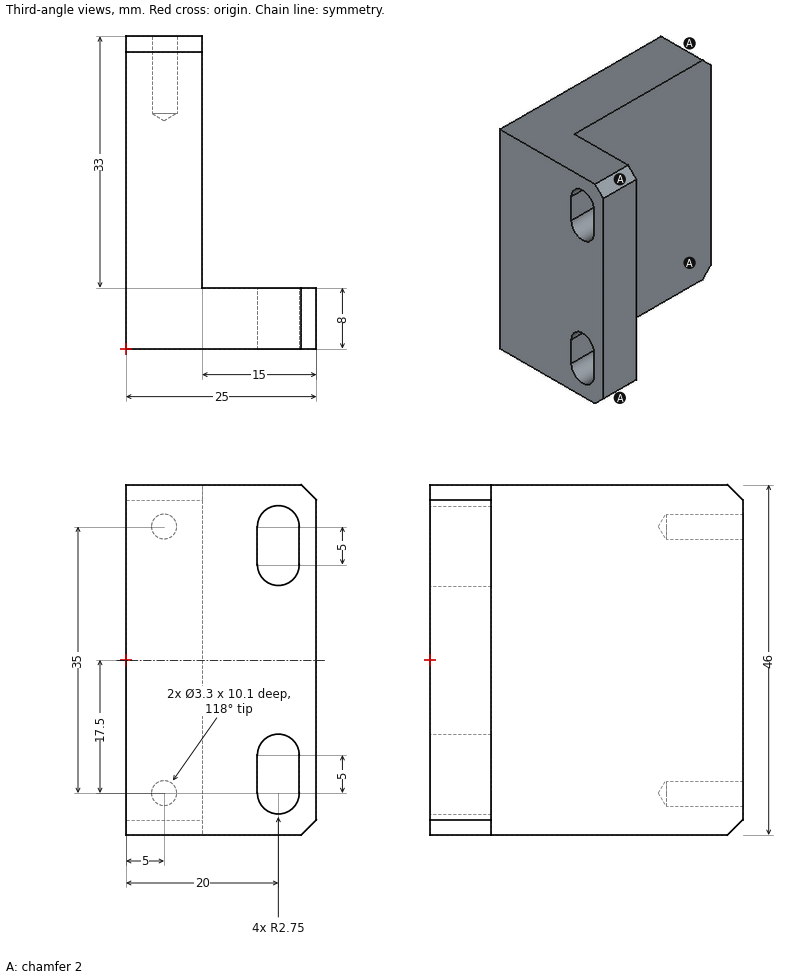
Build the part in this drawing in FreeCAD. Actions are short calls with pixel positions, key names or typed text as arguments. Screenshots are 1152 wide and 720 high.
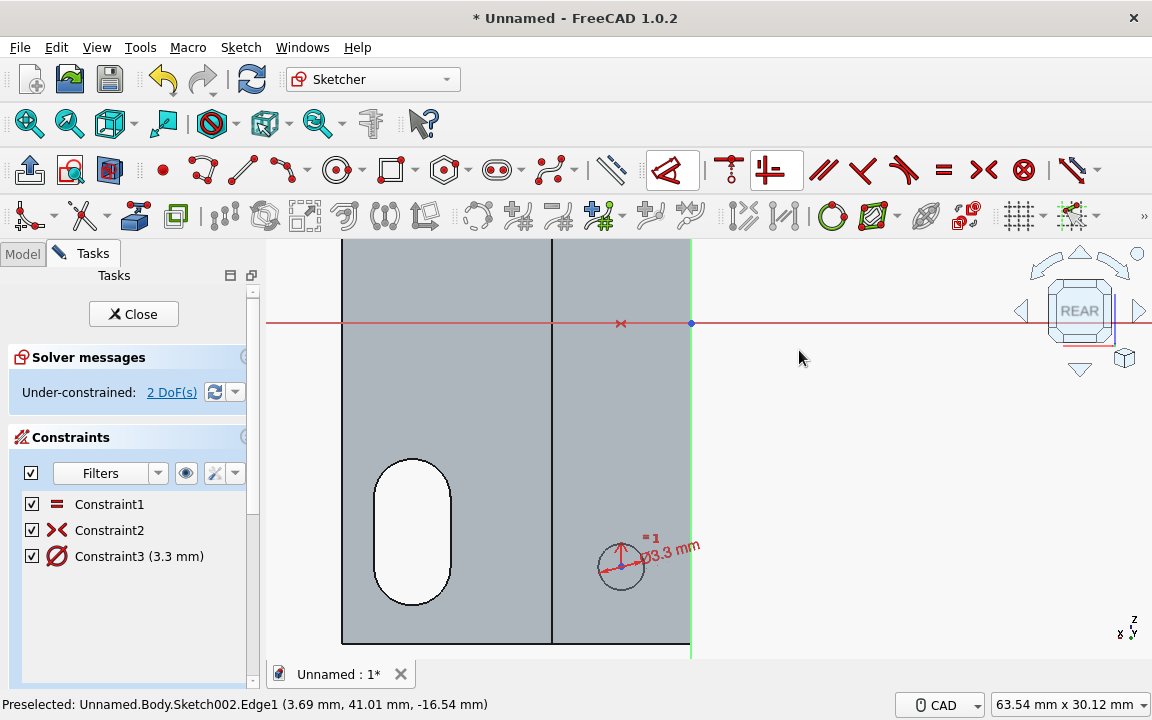
click(621, 567)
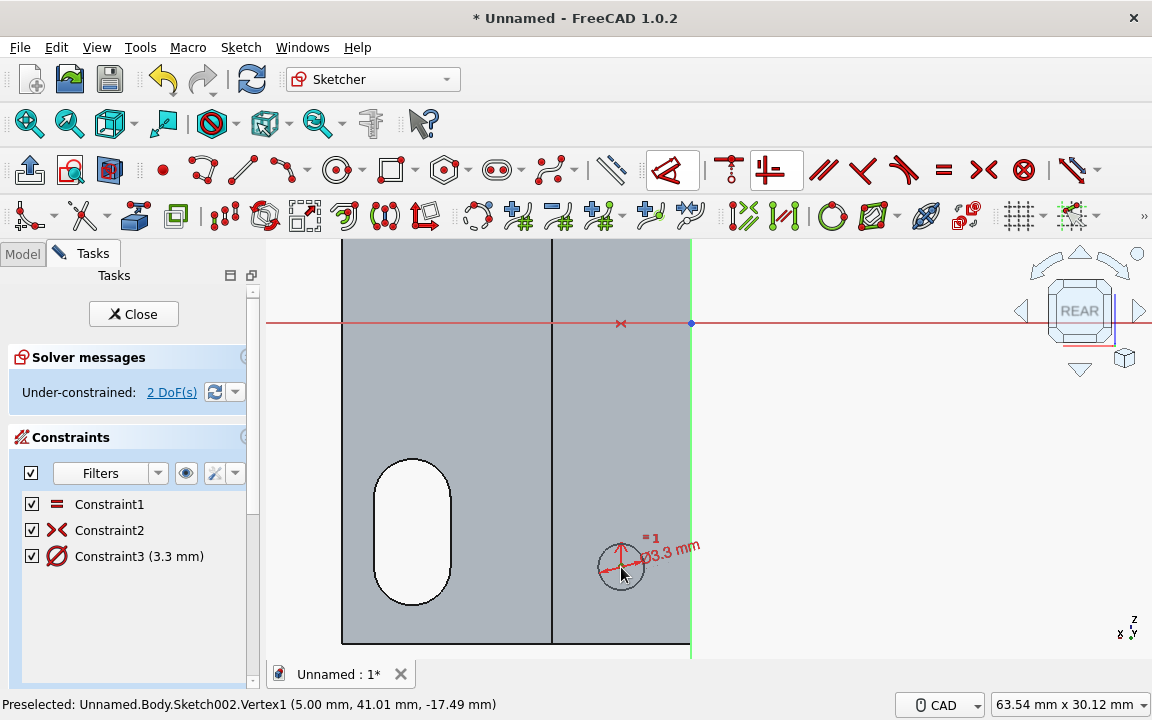
click(694, 170)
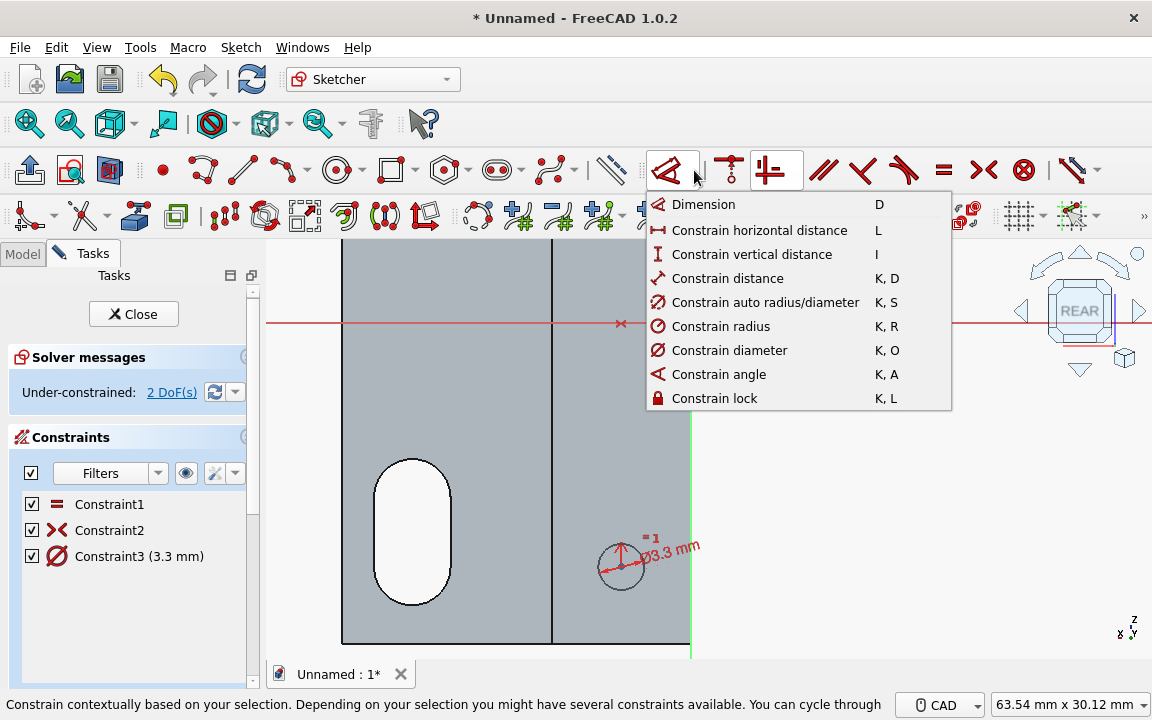
click(799, 230)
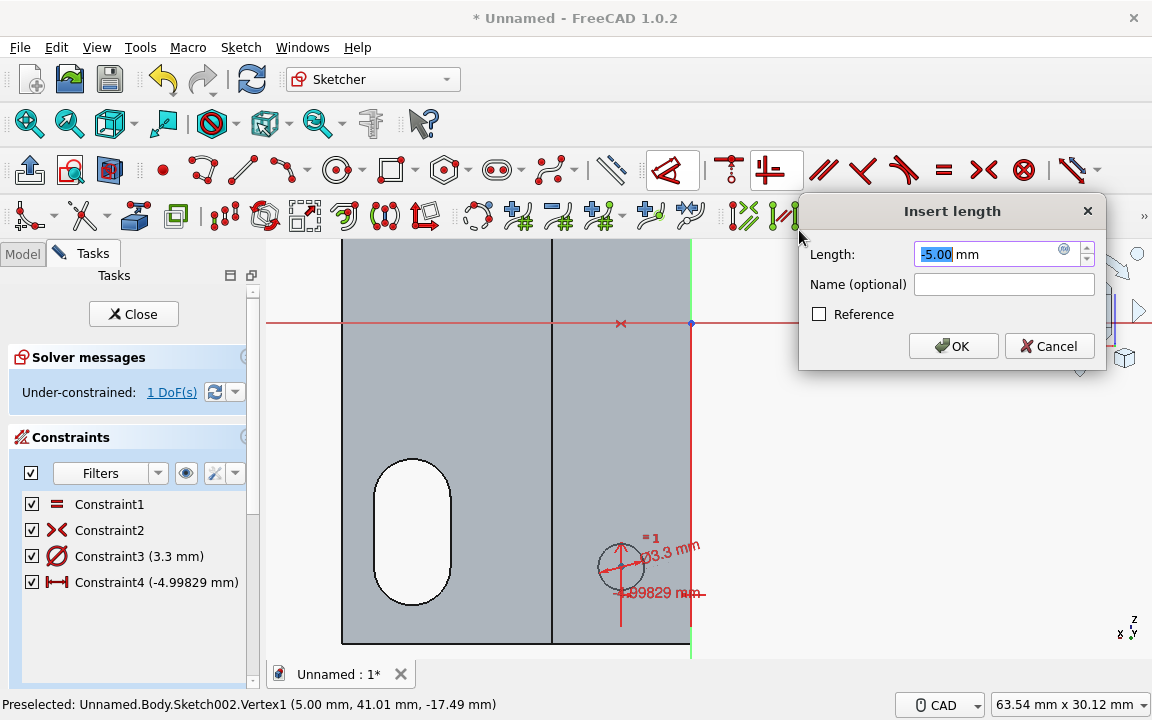
text(-5)
key(Return)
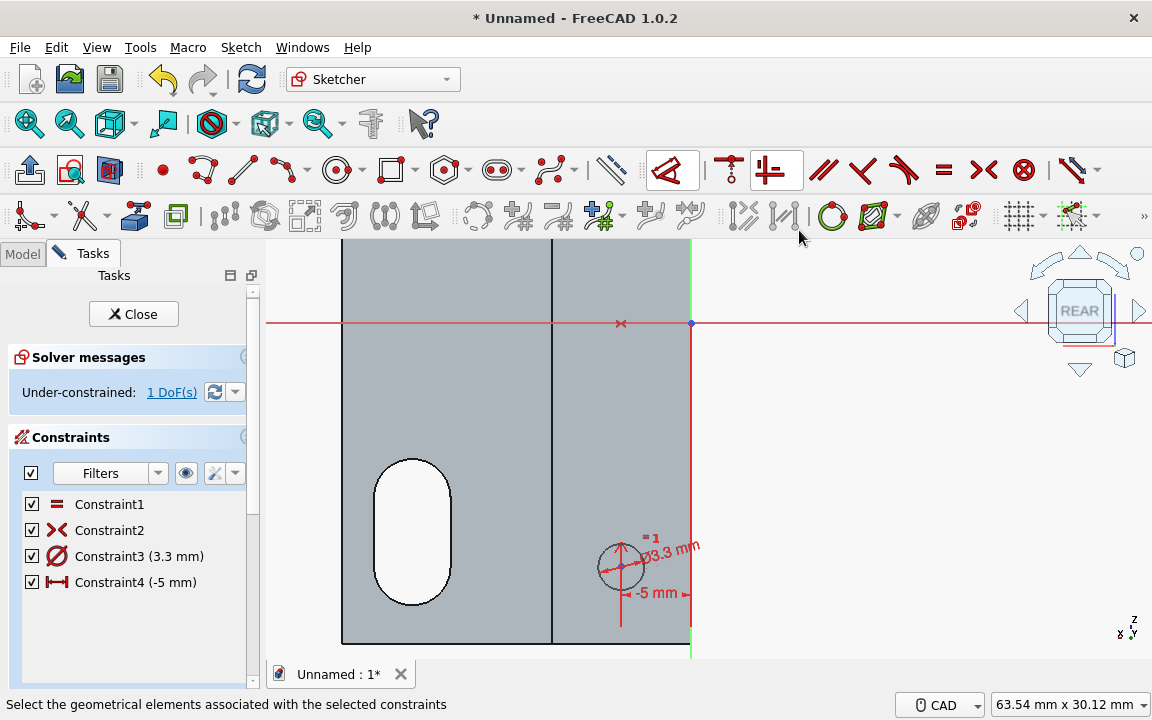
click(621, 567)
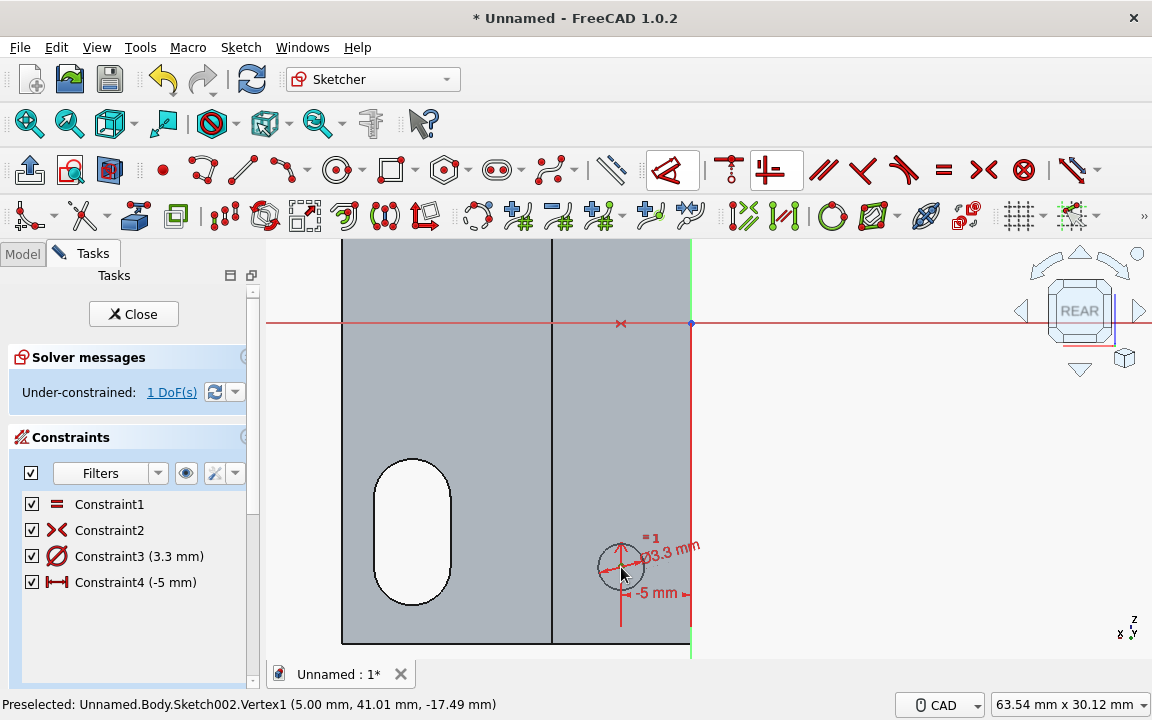
scroll(637, 552, down, 4)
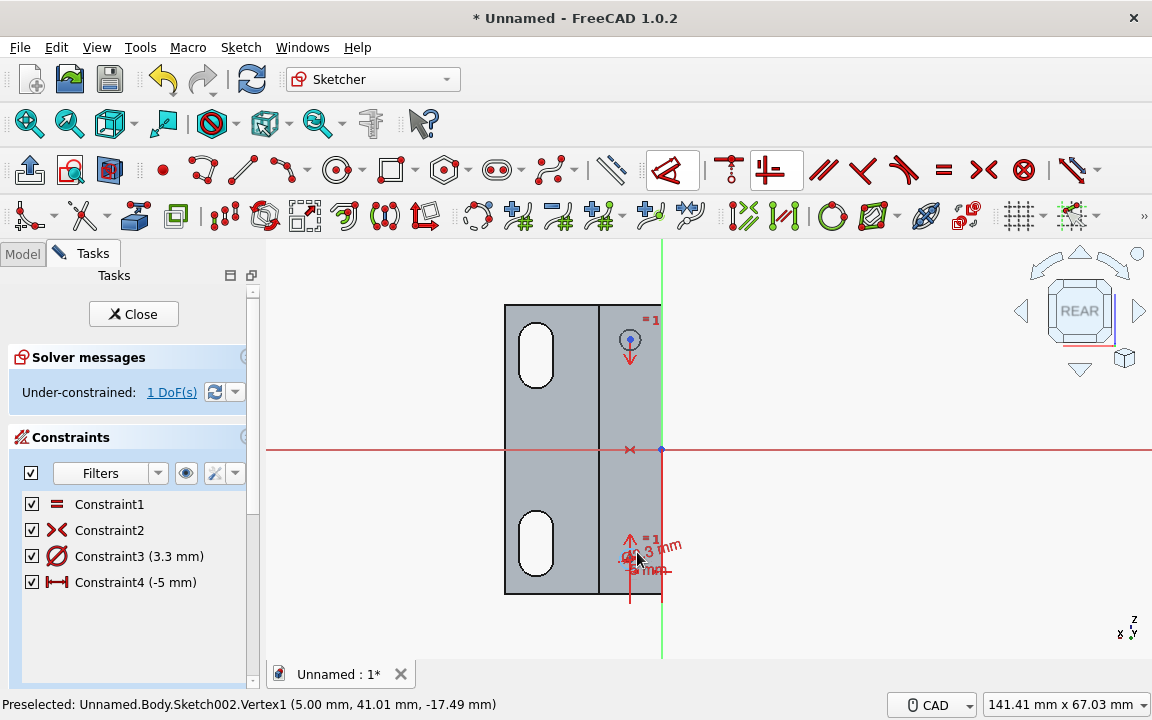
click(630, 340)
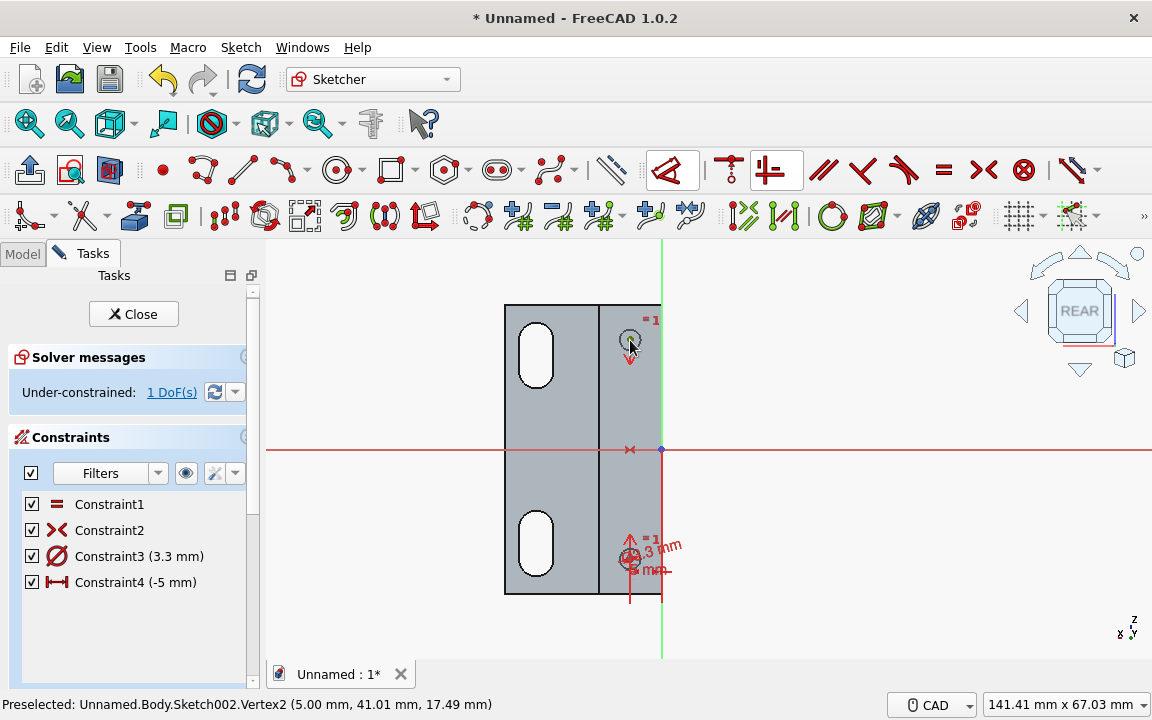
key(i)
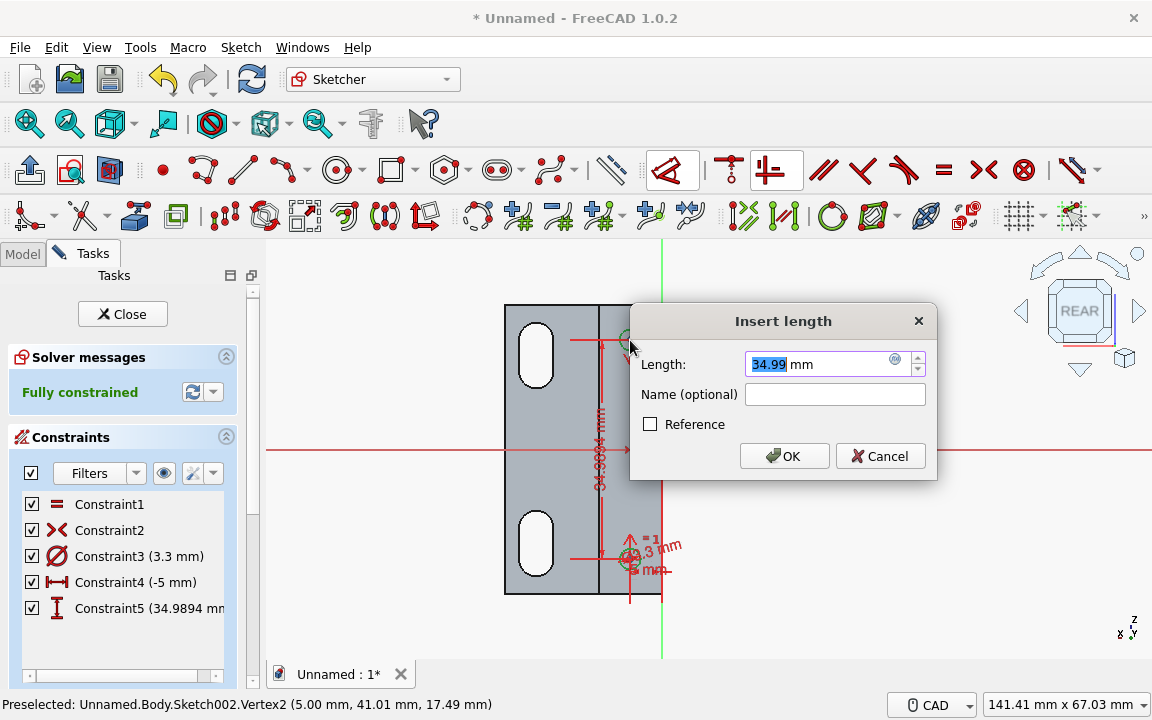
text(35)
key(Return)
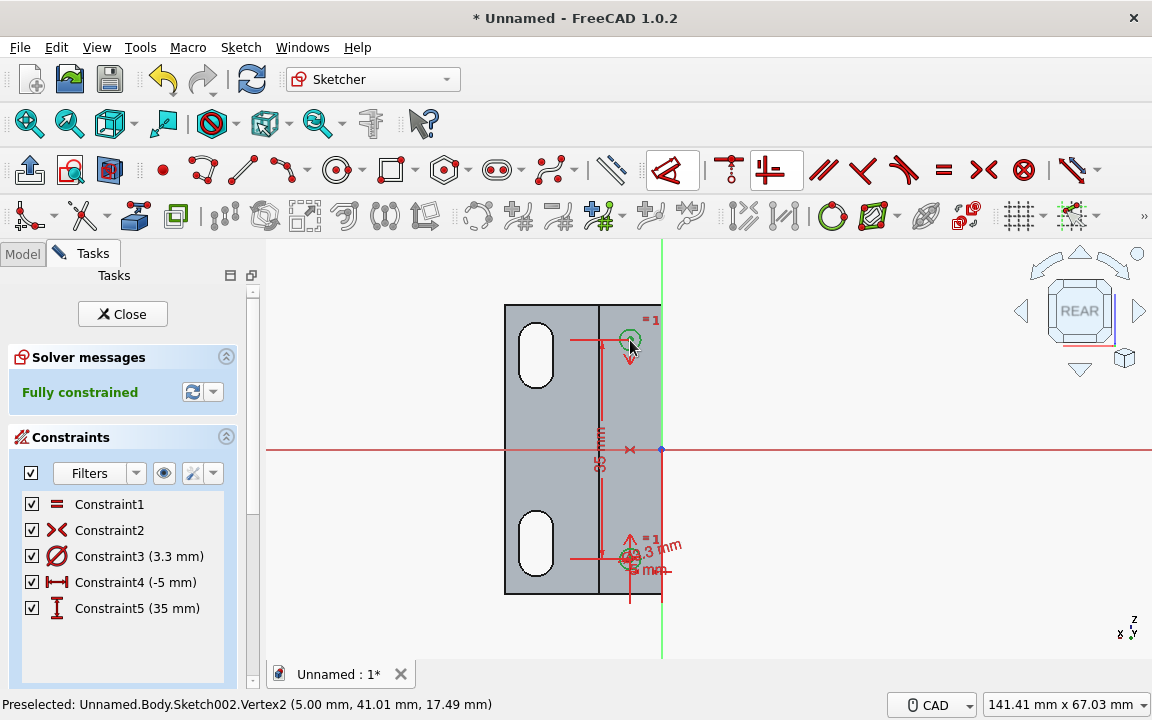
click(123, 314)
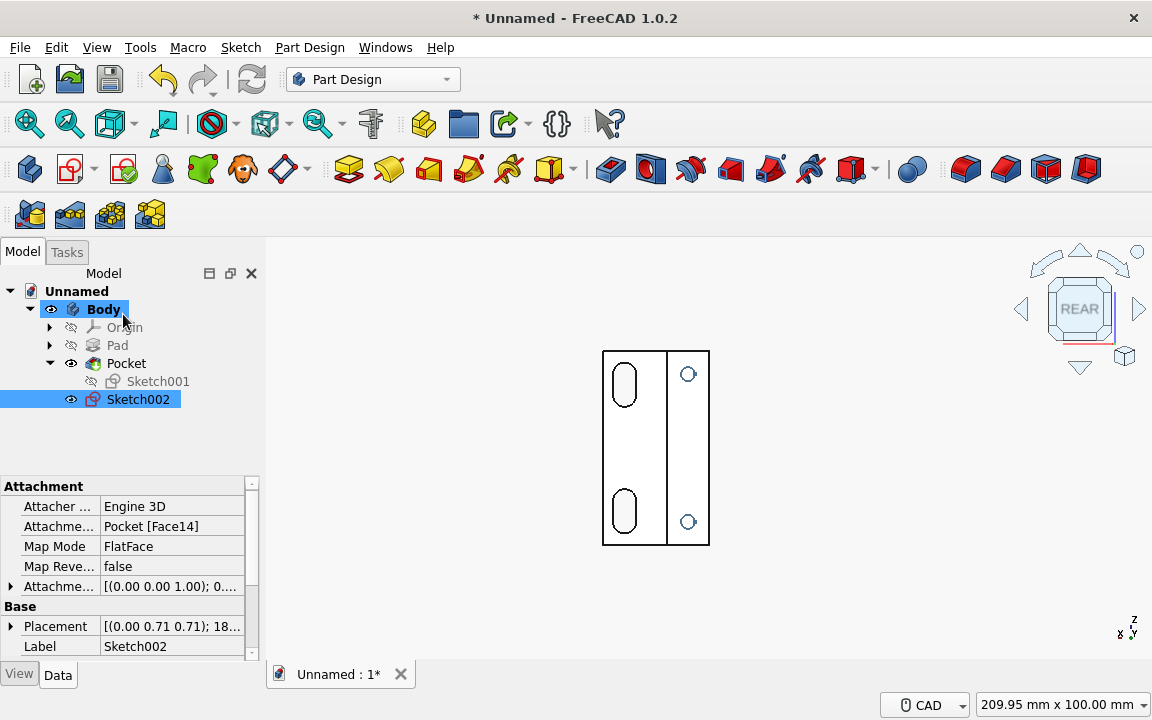
click(652, 170)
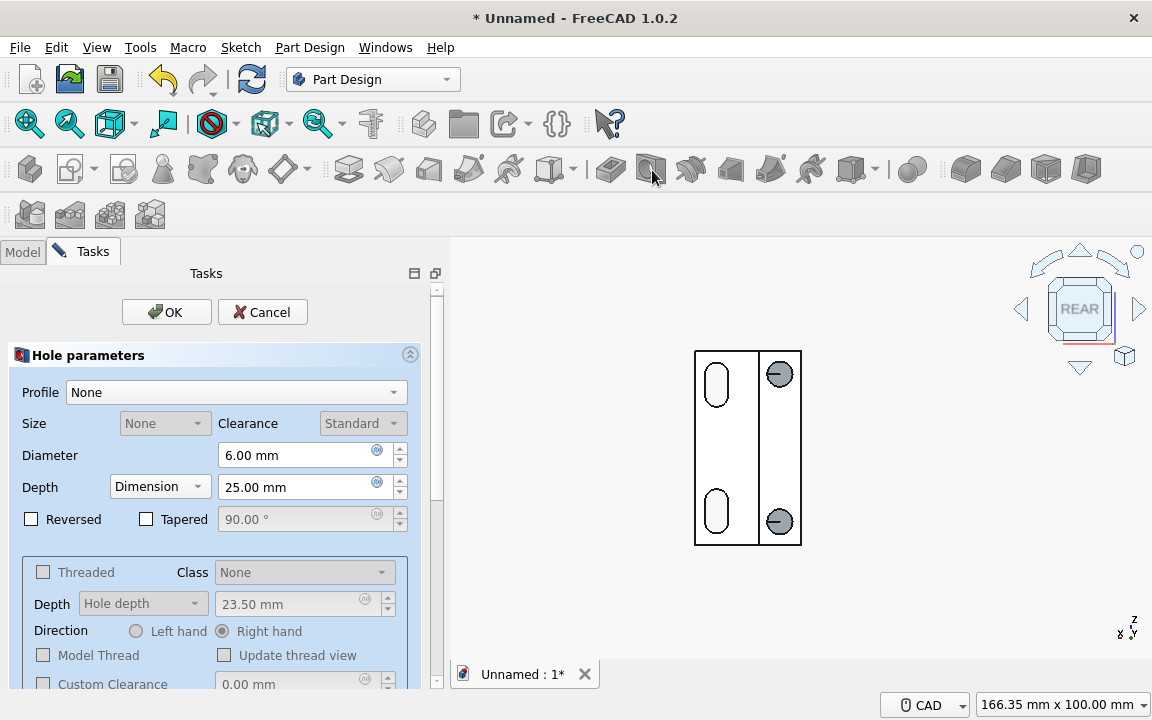
triple_click(305, 455)